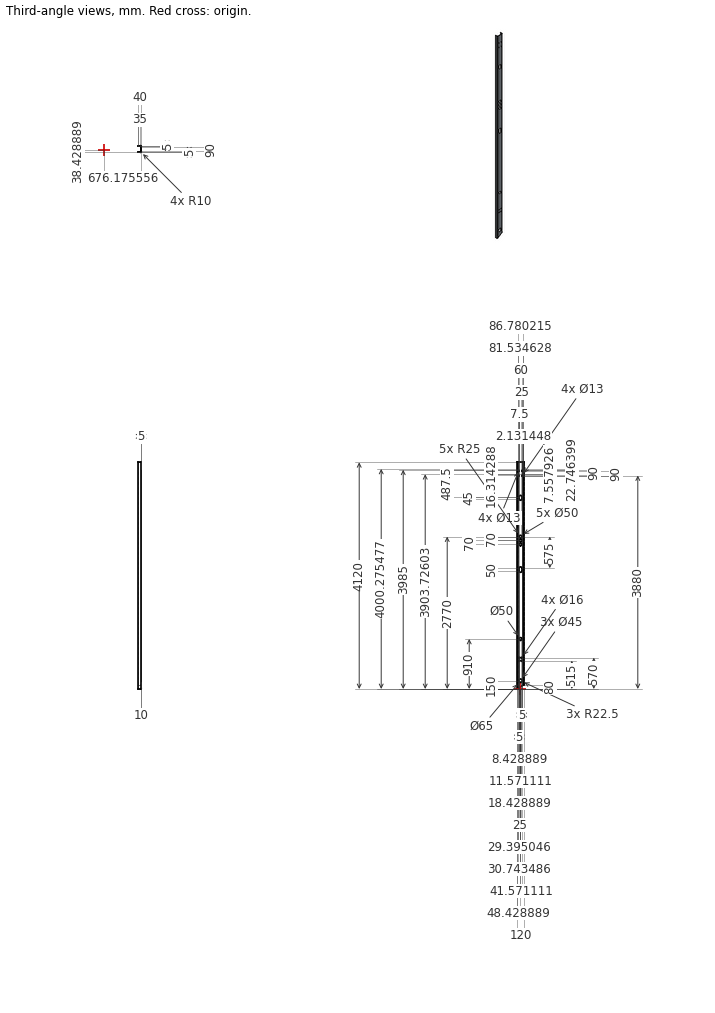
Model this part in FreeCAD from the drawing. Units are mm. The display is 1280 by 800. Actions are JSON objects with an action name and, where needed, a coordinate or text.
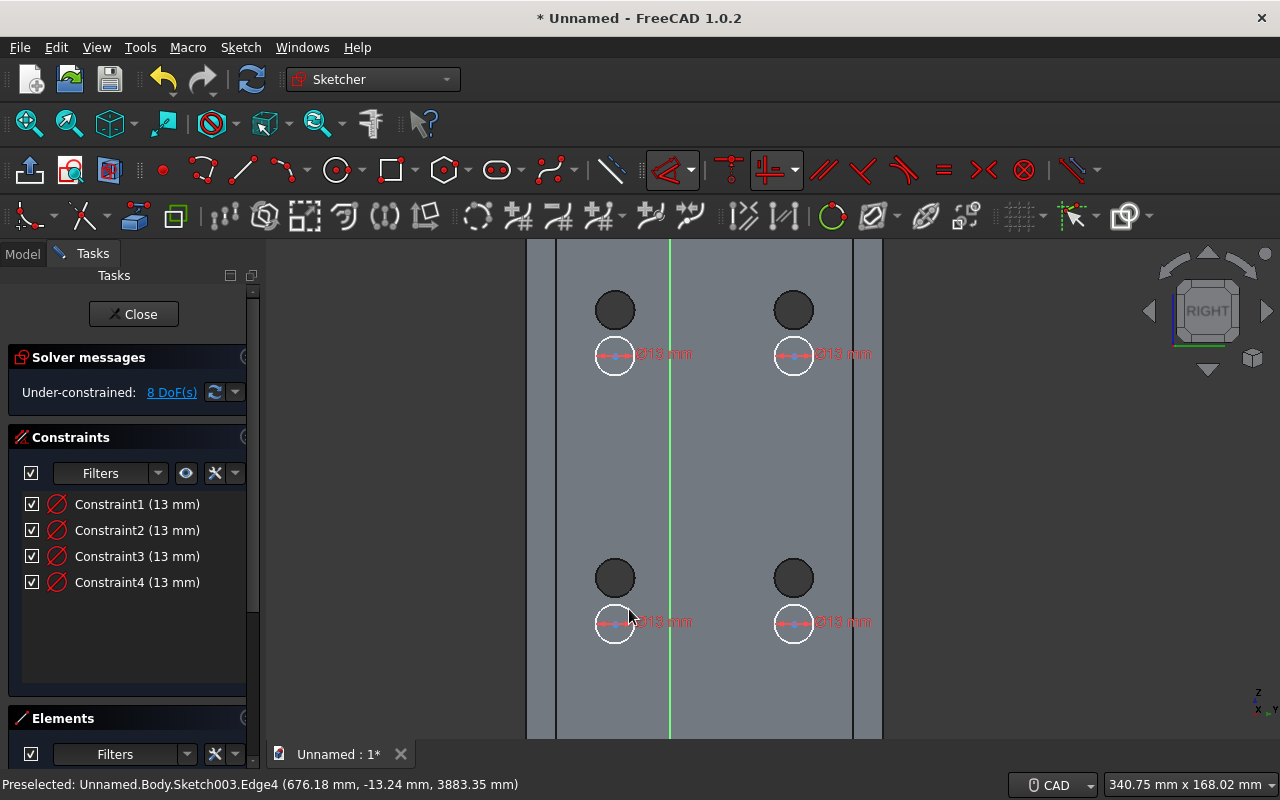
{"action": "left_click", "coordinate": [794, 624]}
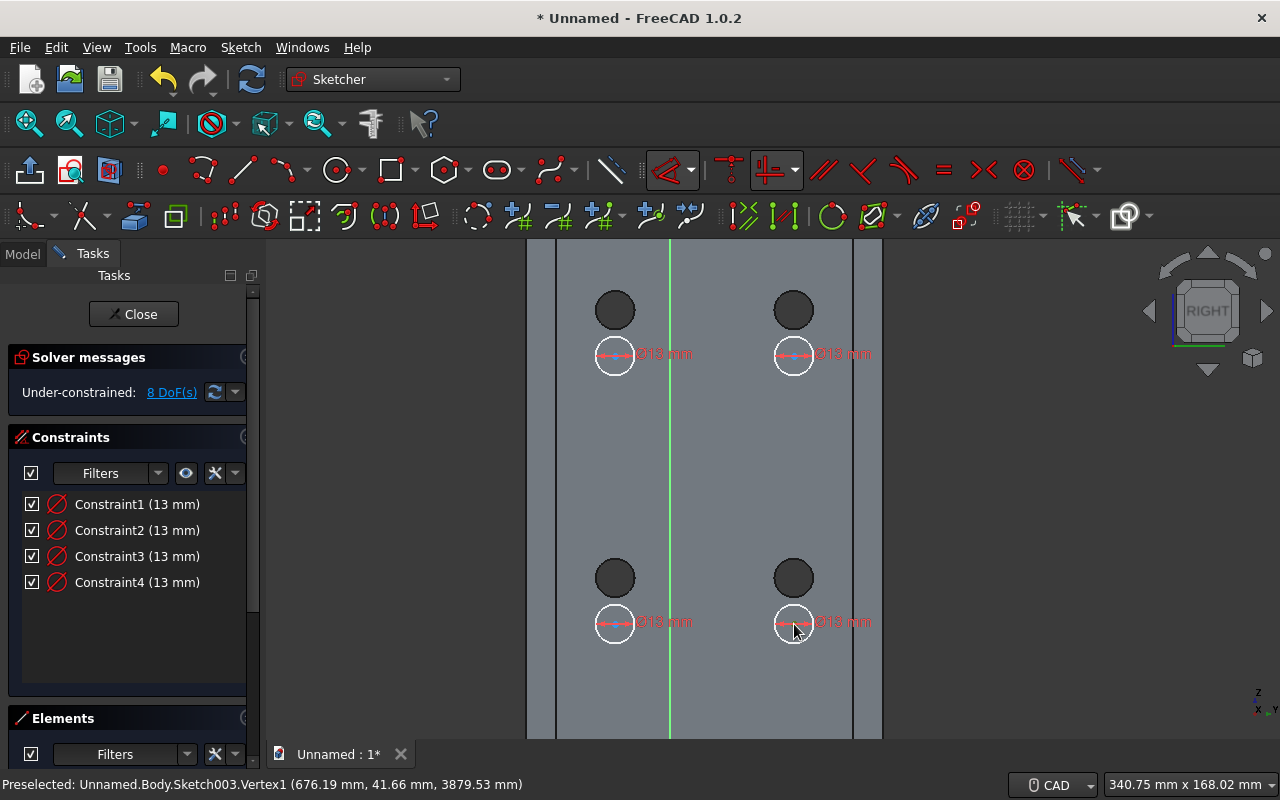
{"action": "left_click", "coordinate": [794, 356]}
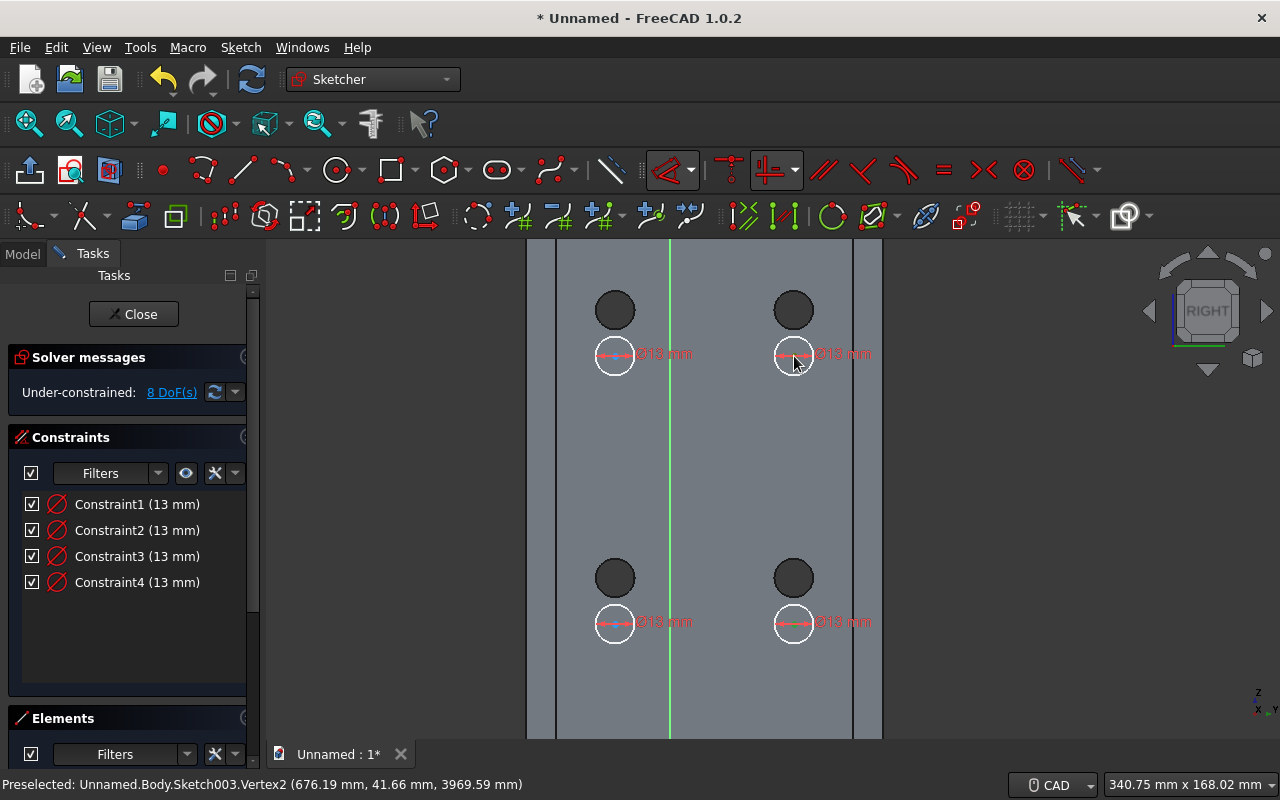
{"action": "key", "text": "v"}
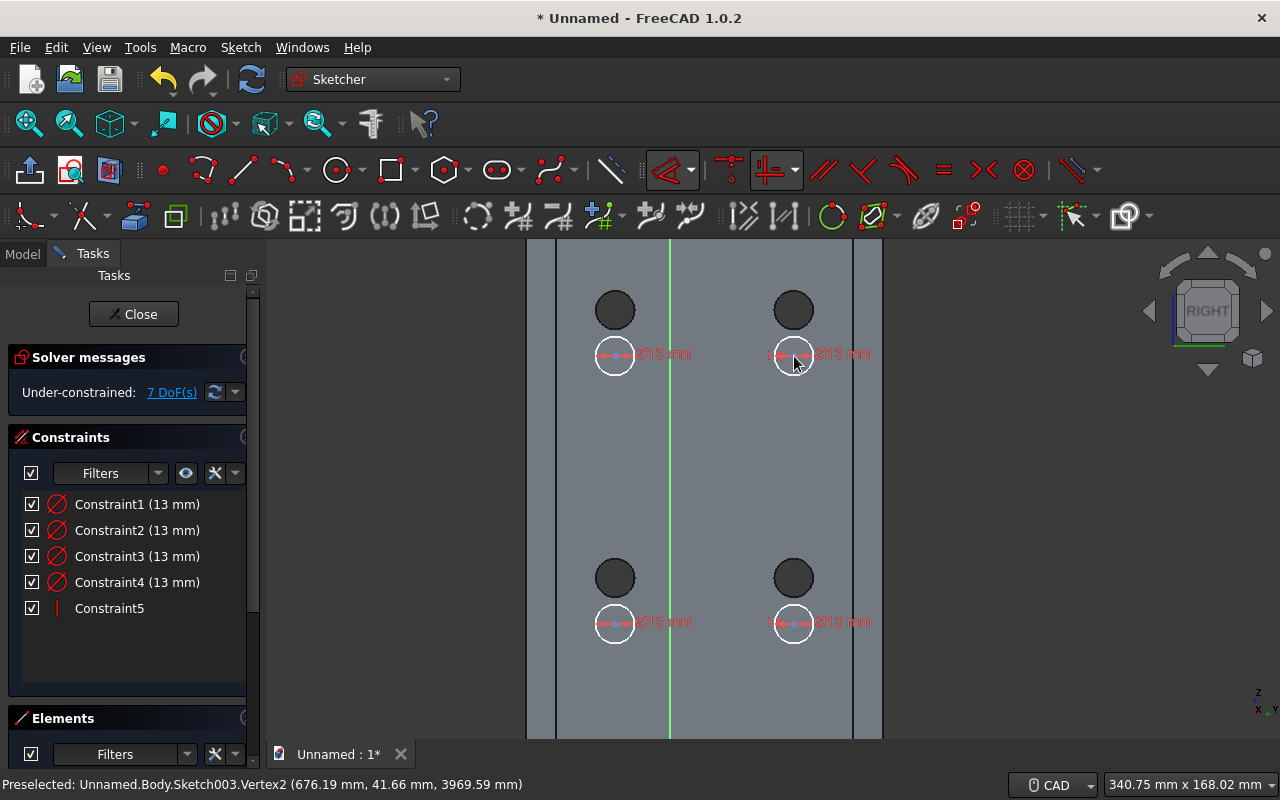
{"action": "left_click", "coordinate": [794, 356]}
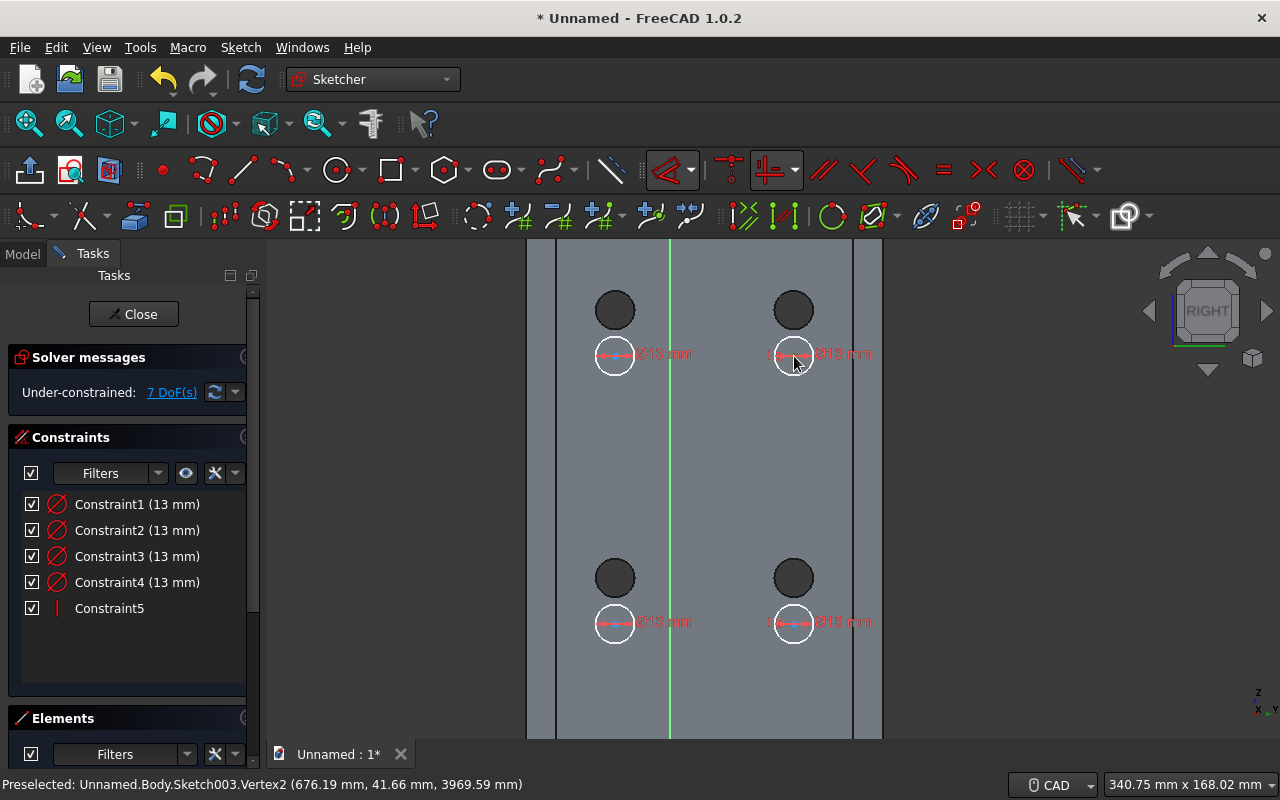
{"action": "left_click", "coordinate": [615, 356]}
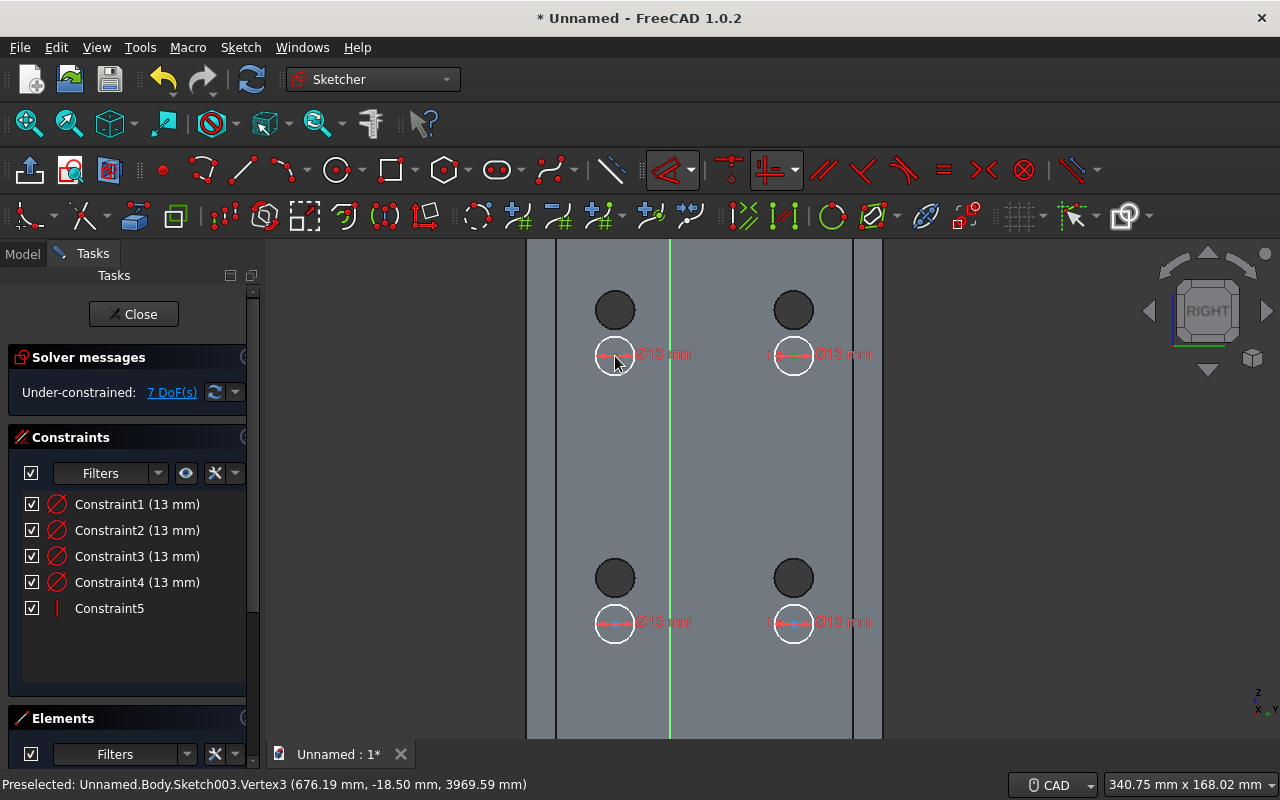
{"action": "key", "text": "h"}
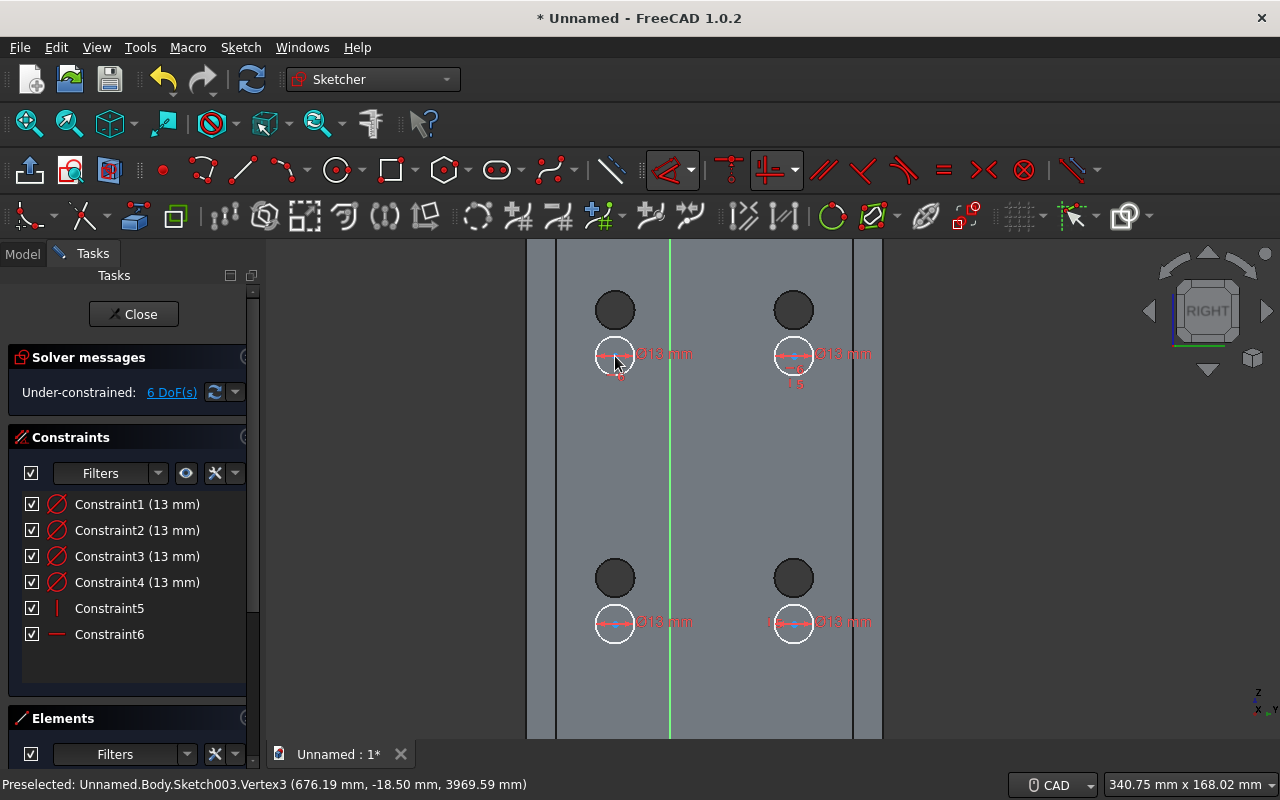
{"action": "left_click", "coordinate": [615, 356]}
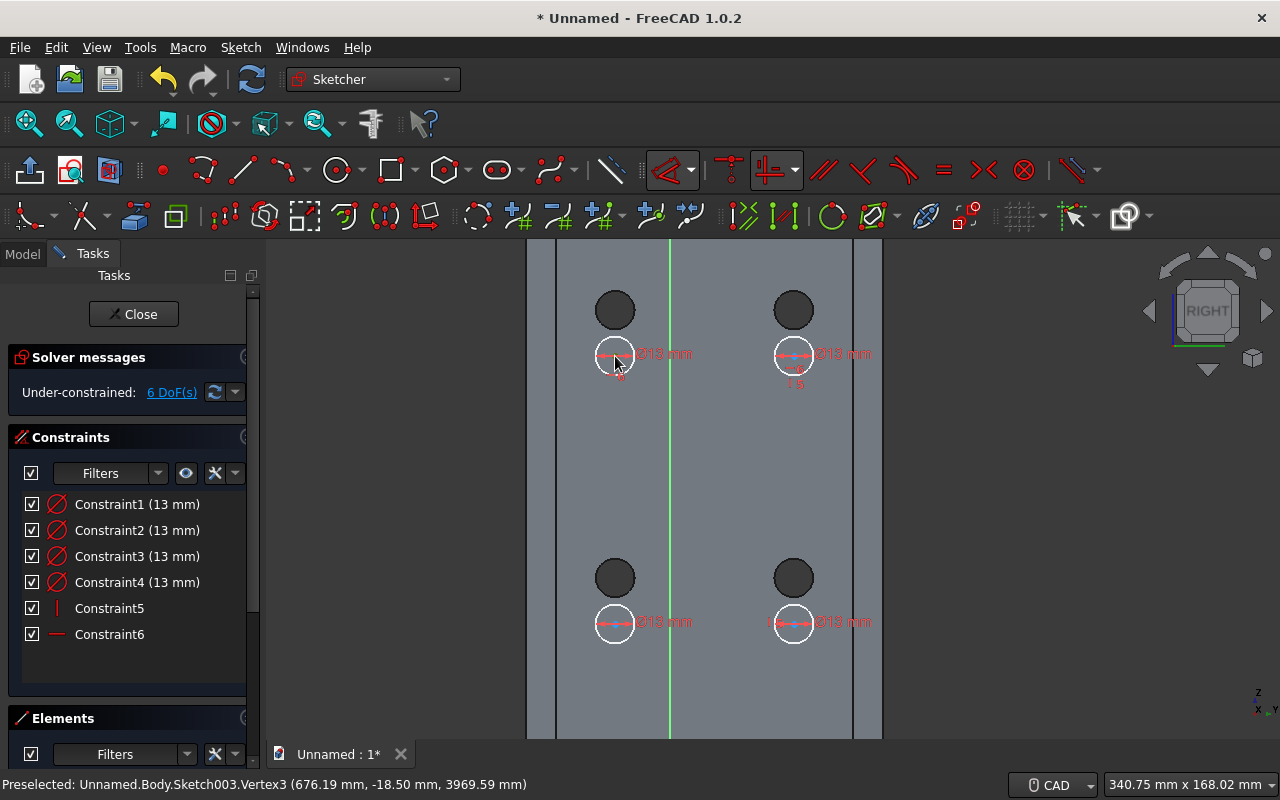
{"action": "left_click", "coordinate": [615, 624]}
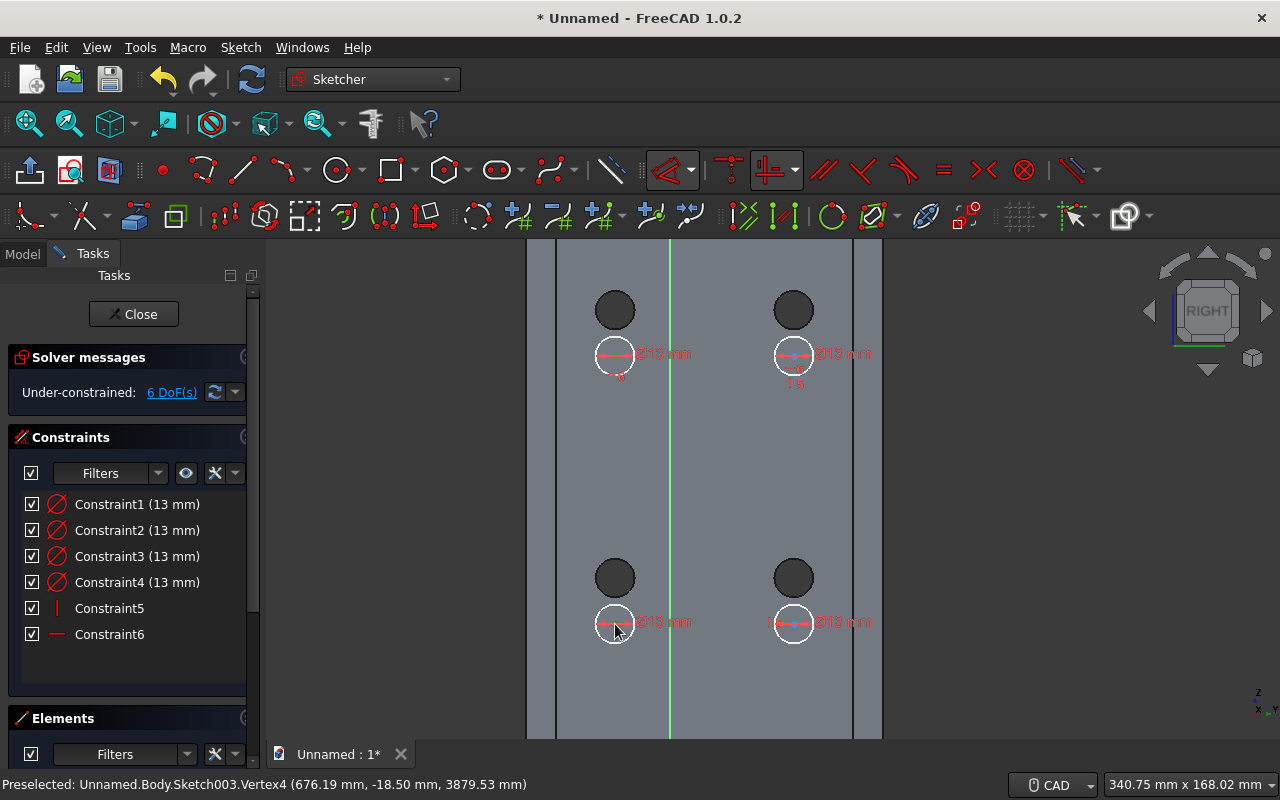
{"action": "key", "text": "v"}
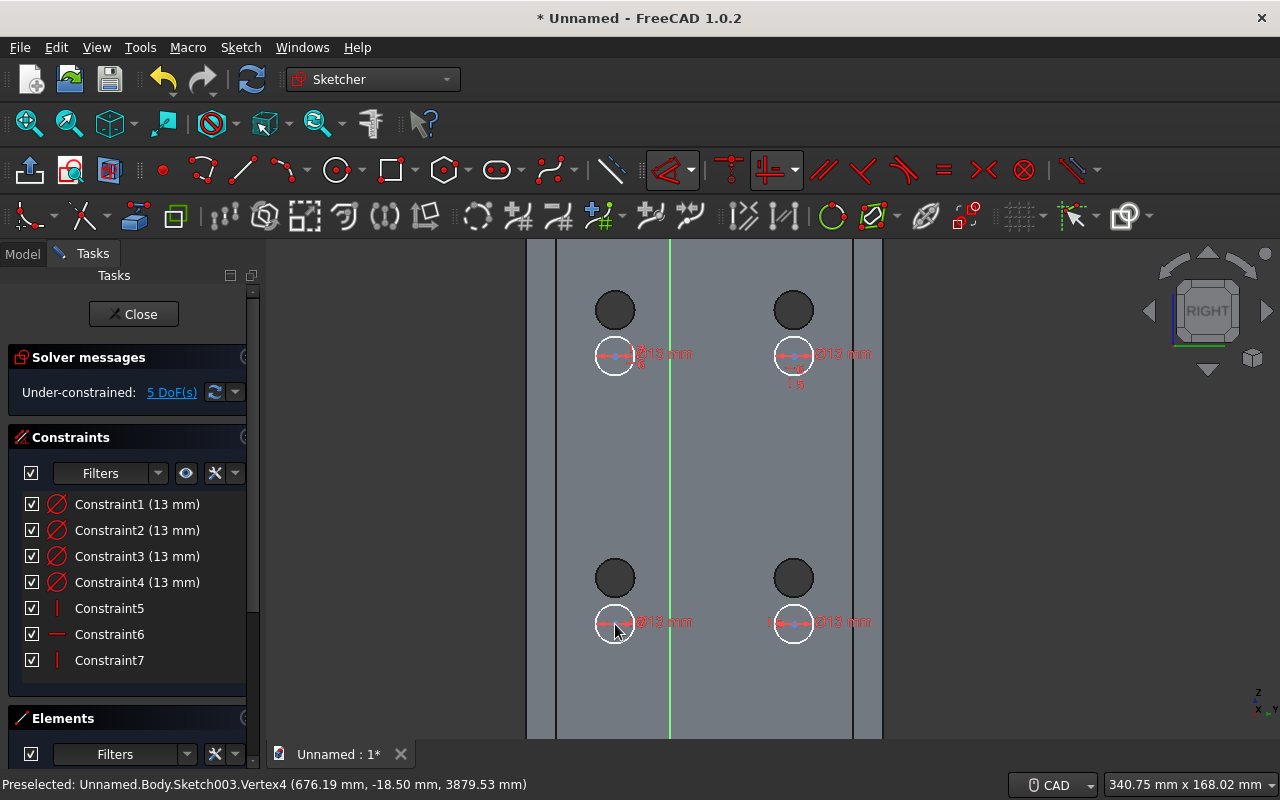
{"action": "left_click", "coordinate": [794, 624]}